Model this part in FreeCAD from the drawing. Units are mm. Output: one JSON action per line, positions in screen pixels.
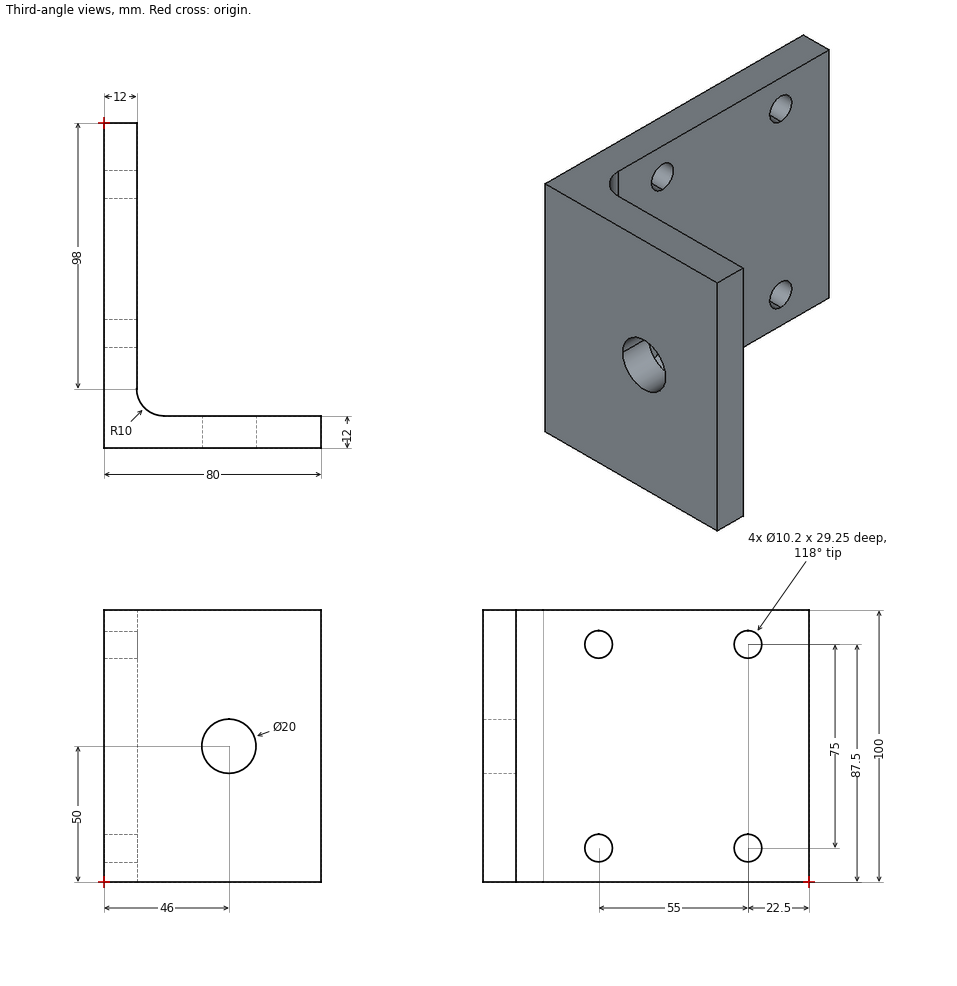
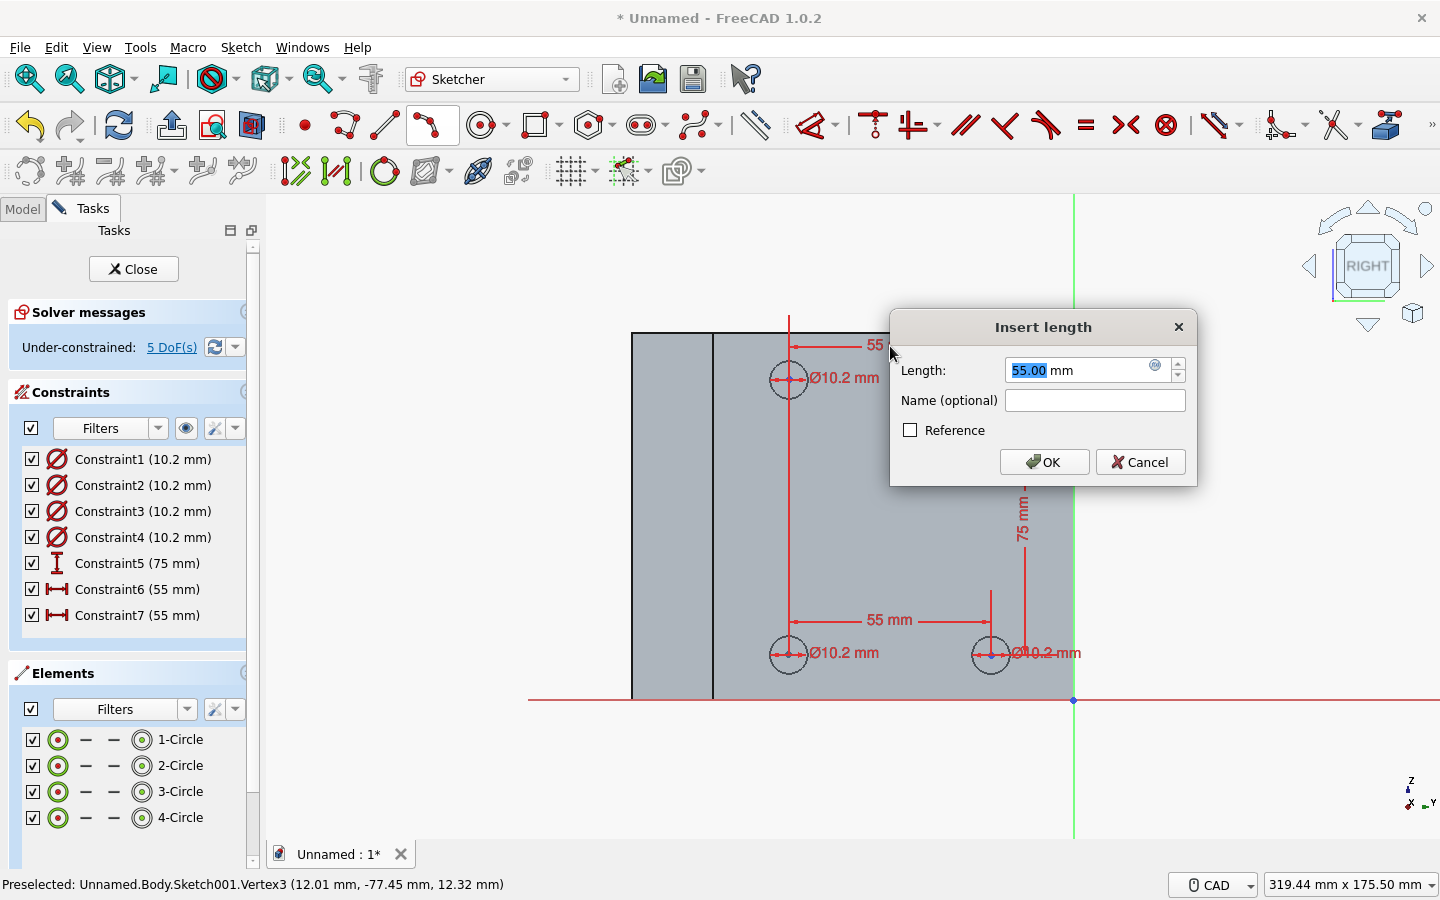
{"action": "type", "text": "55"}
{"action": "key", "text": "Return"}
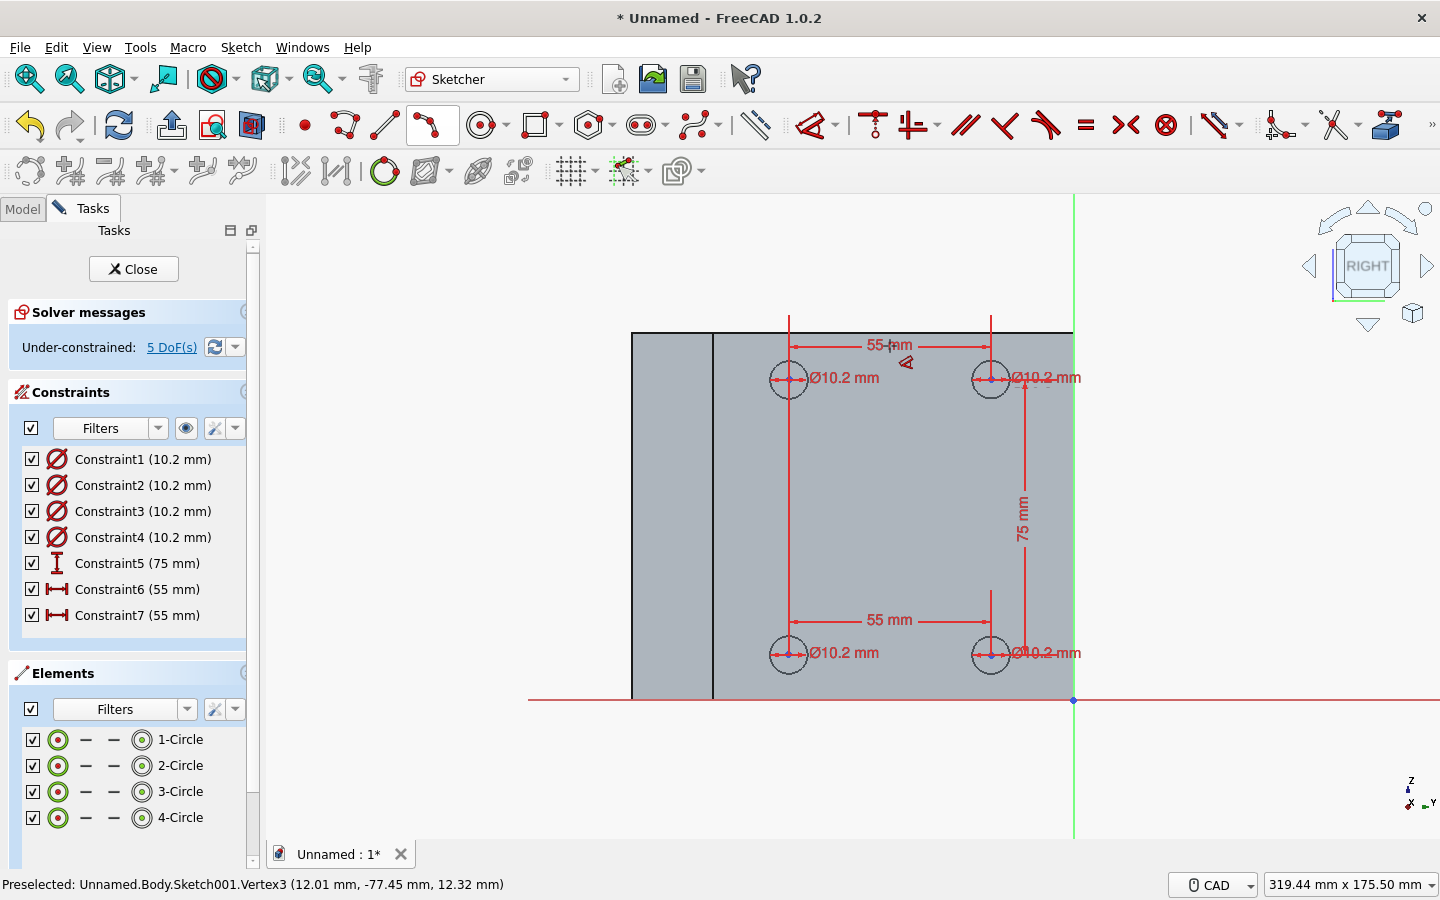
{"action": "left_click", "coordinate": [991, 380]}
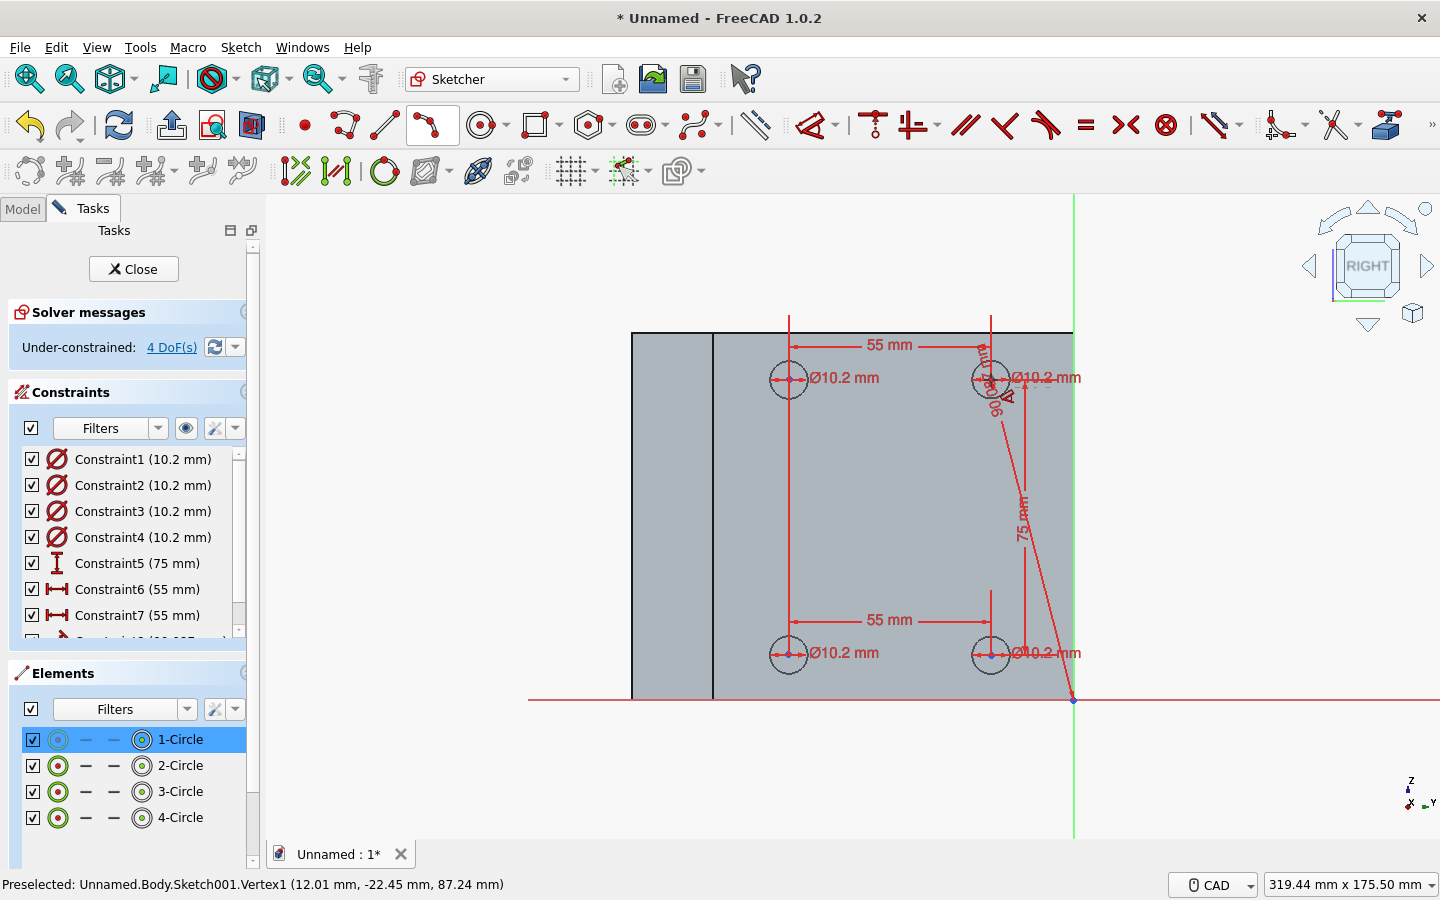
{"action": "left_click", "coordinate": [789, 655]}
{"action": "left_click", "coordinate": [755, 517]}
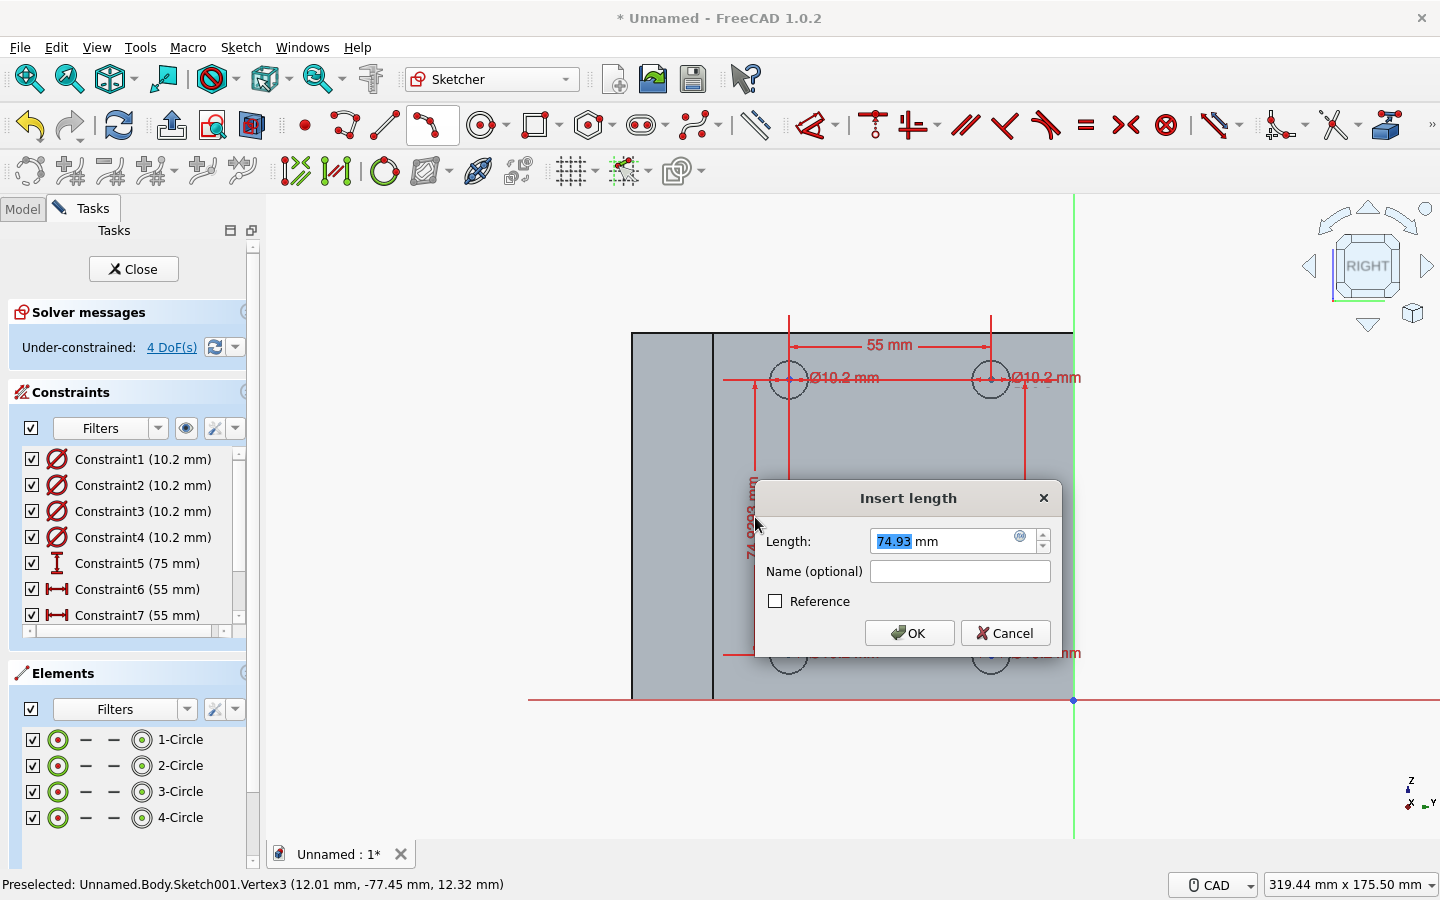
{"action": "type", "text": "75"}
{"action": "key", "text": "Return"}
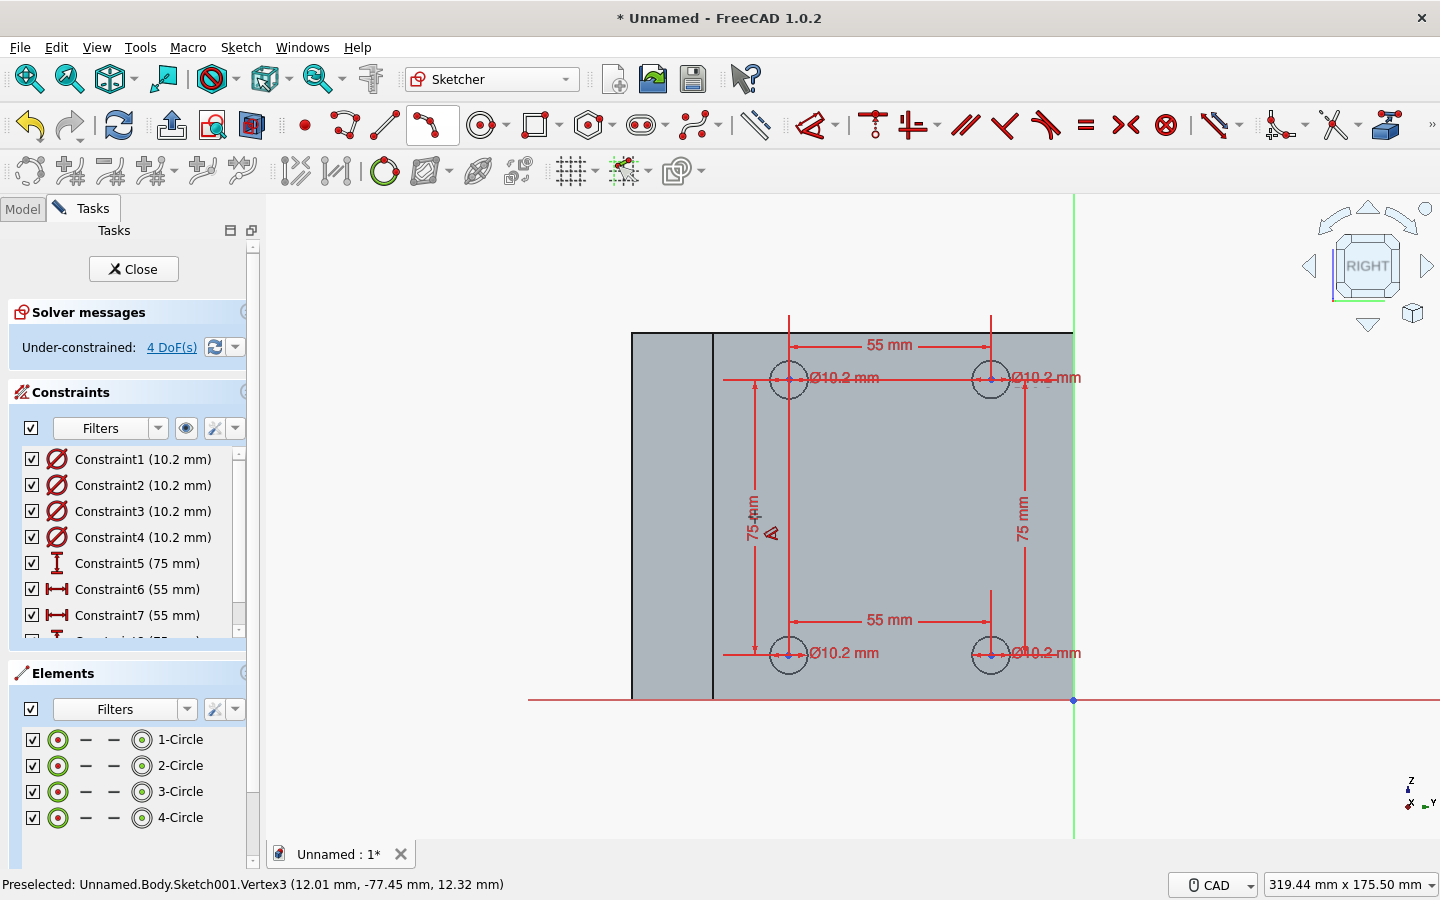
{"action": "left_click", "coordinate": [991, 380]}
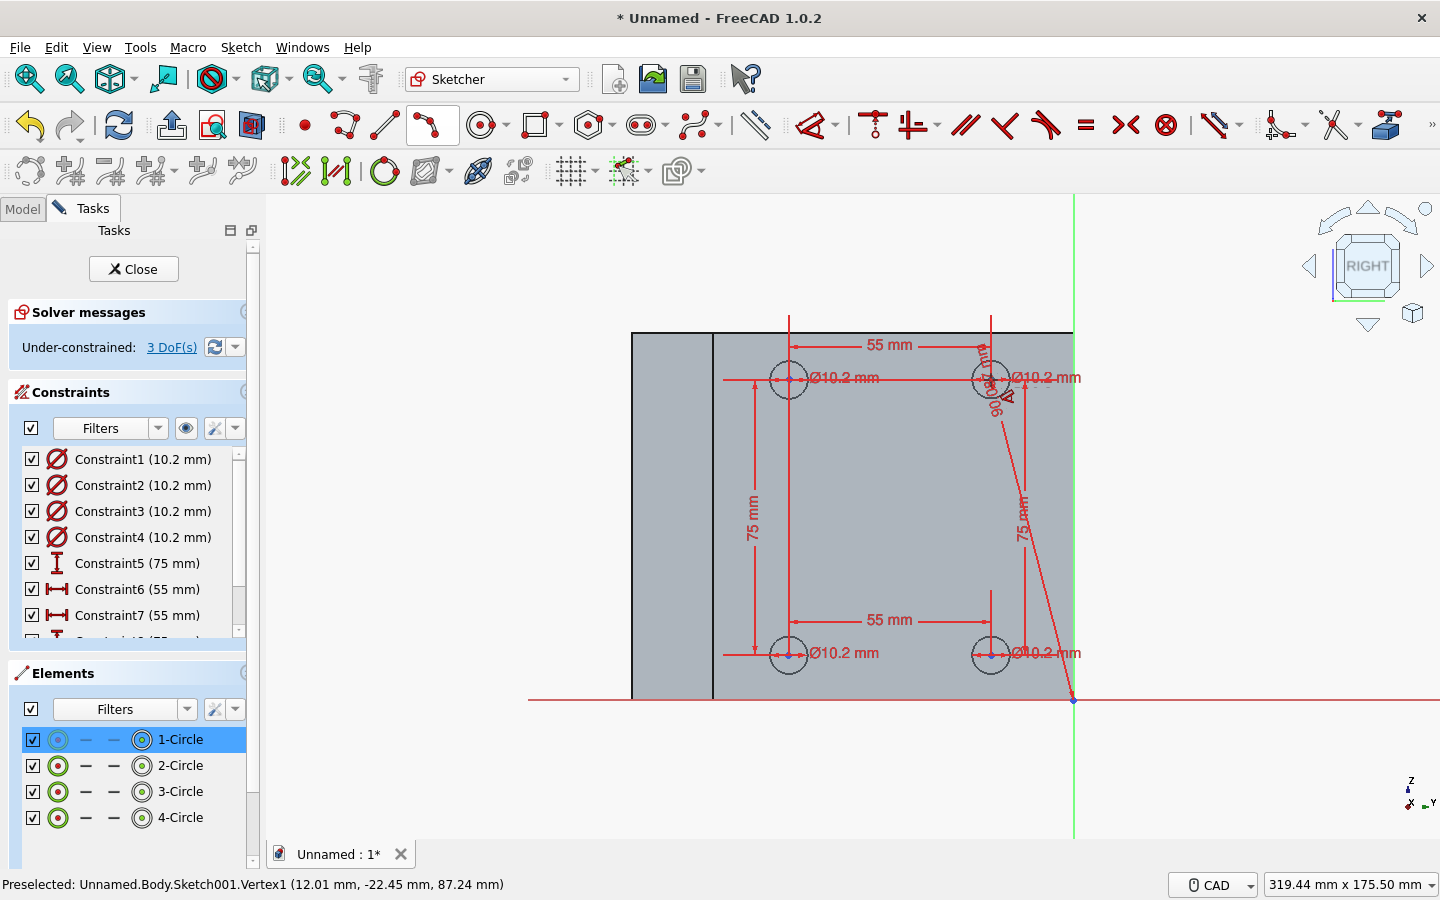
{"action": "left_click", "coordinate": [789, 380]}
{"action": "left_click", "coordinate": [819, 346]}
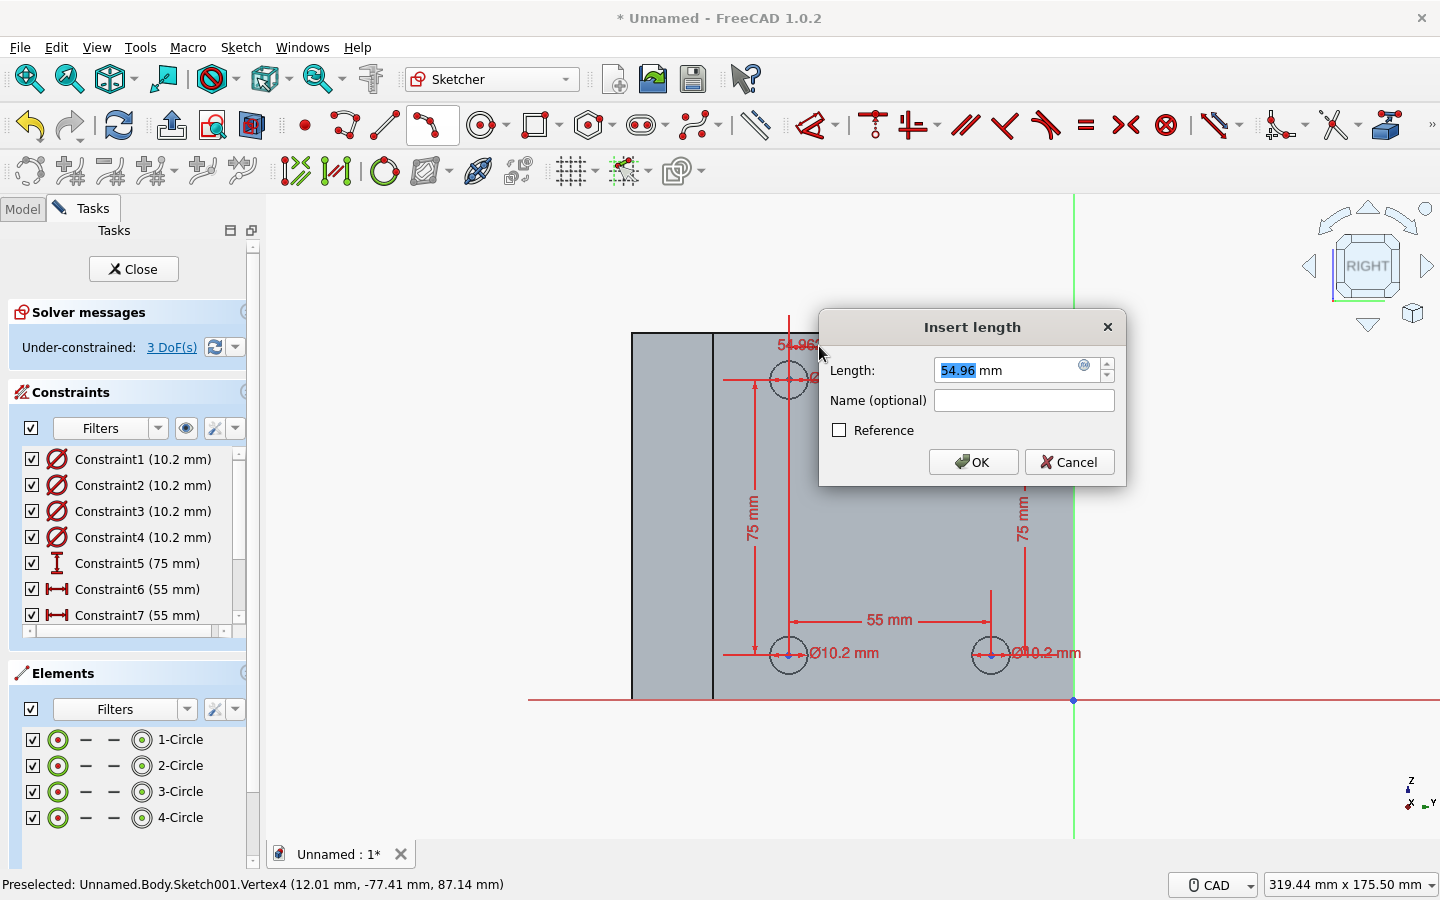
{"action": "type", "text": "55"}
{"action": "key", "text": "Return"}